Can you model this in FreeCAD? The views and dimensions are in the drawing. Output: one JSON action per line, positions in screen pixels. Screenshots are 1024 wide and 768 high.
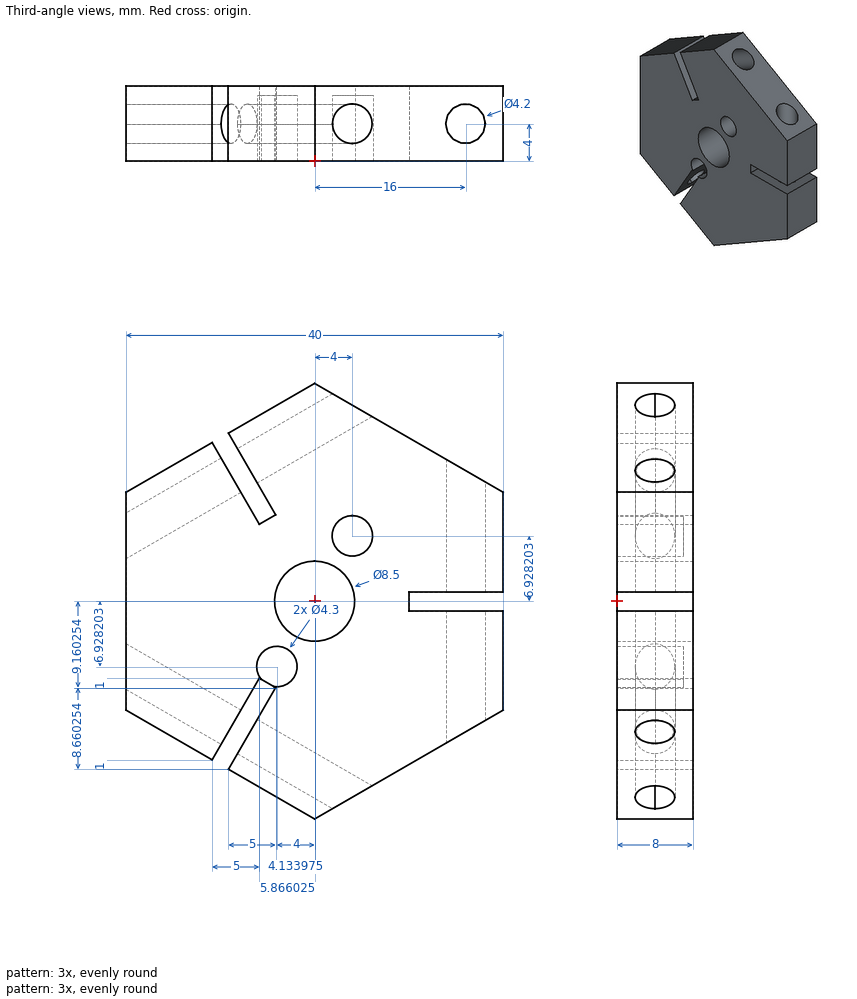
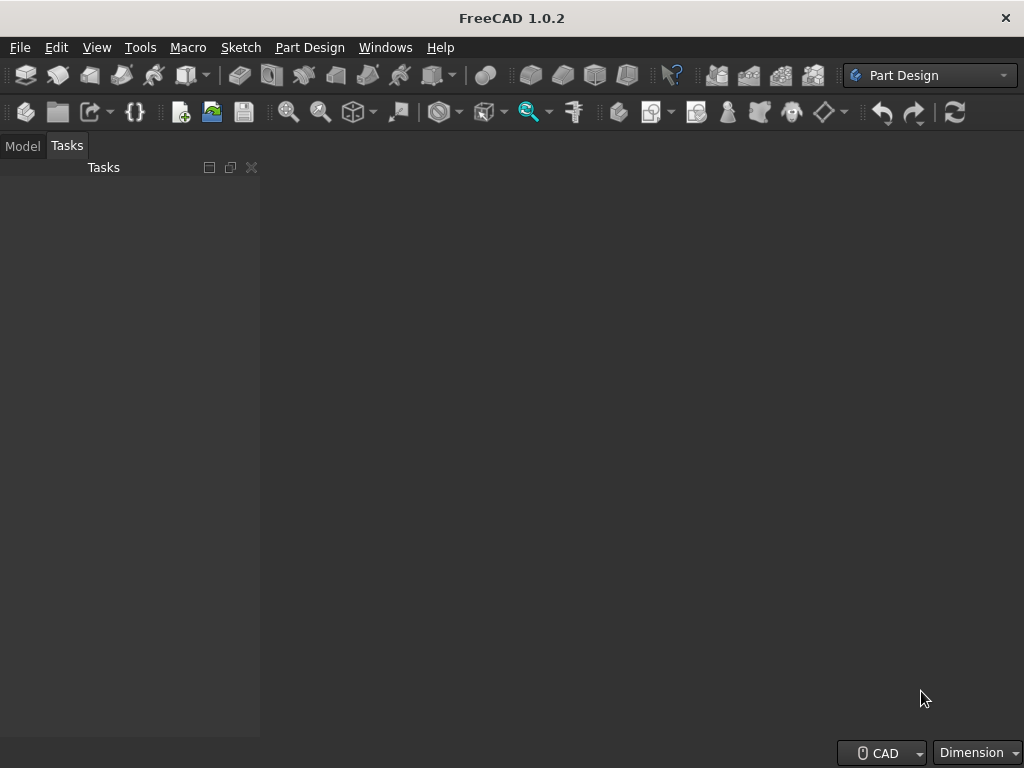
{"action": "left_click", "coordinate": [180, 112]}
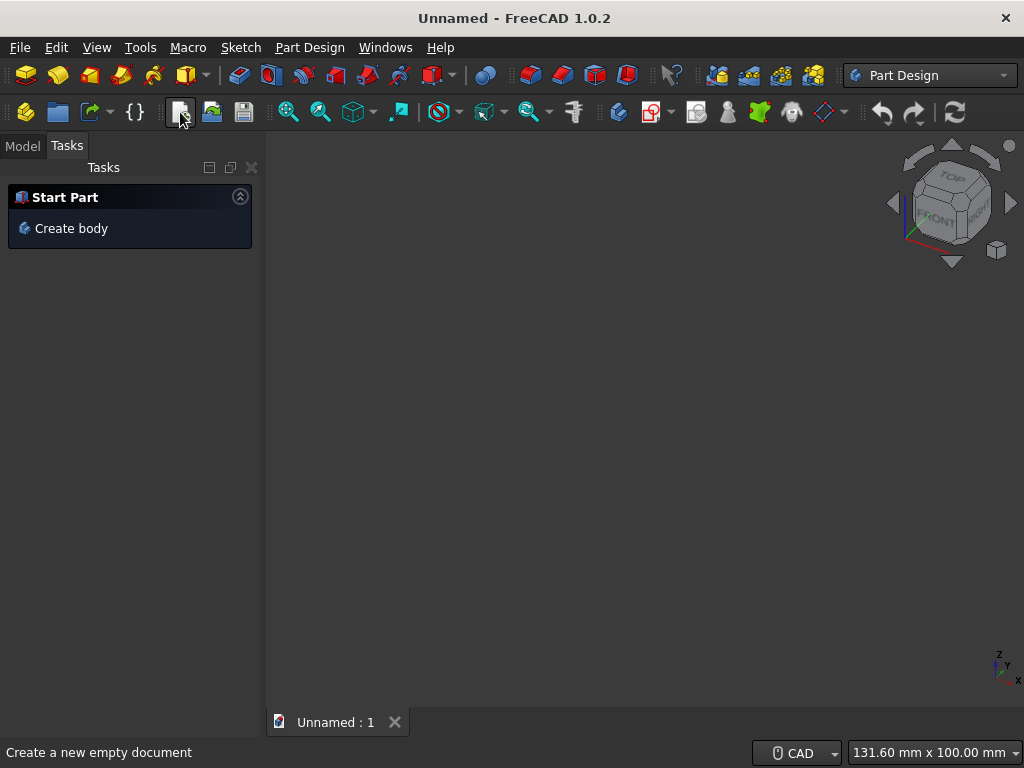
{"action": "left_click", "coordinate": [652, 112]}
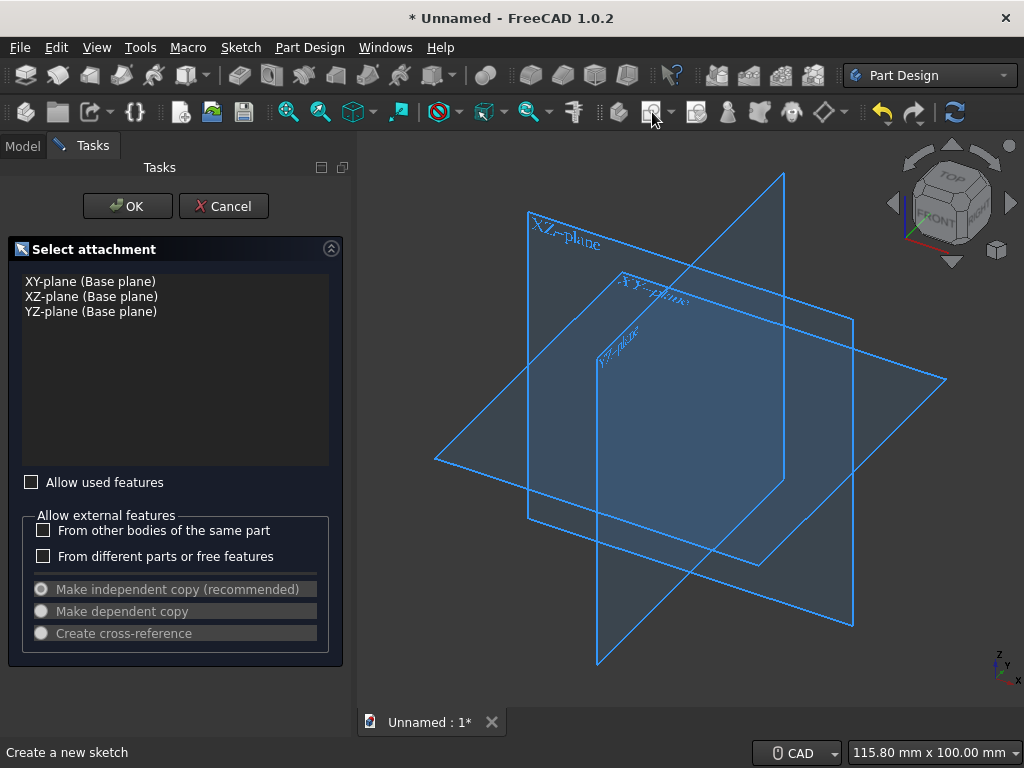
{"action": "left_click", "coordinate": [82, 296]}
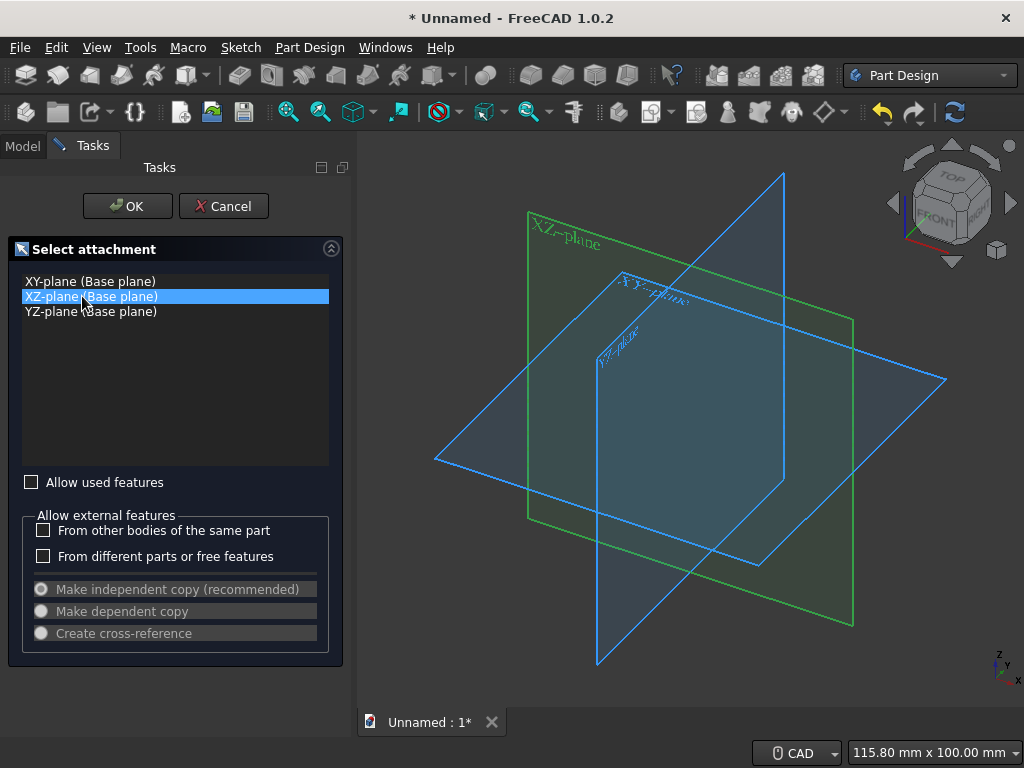
{"action": "left_click", "coordinate": [128, 206]}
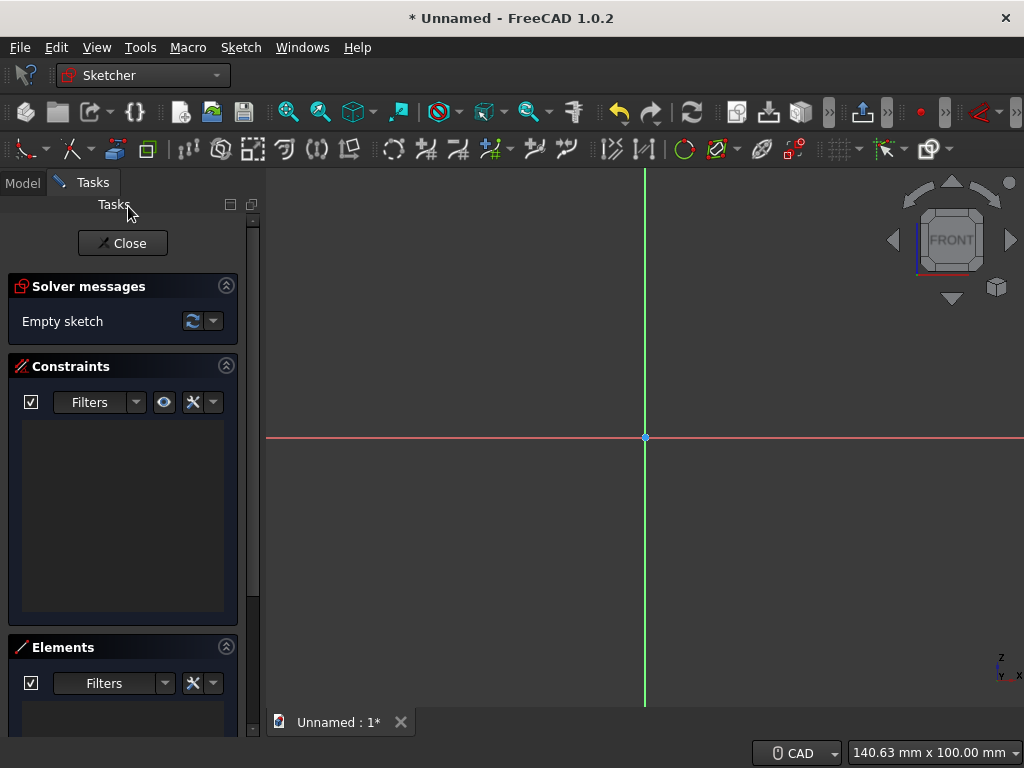
{"action": "scroll", "coordinate": [784, 438], "scroll_direction": "up", "scroll_amount": 2}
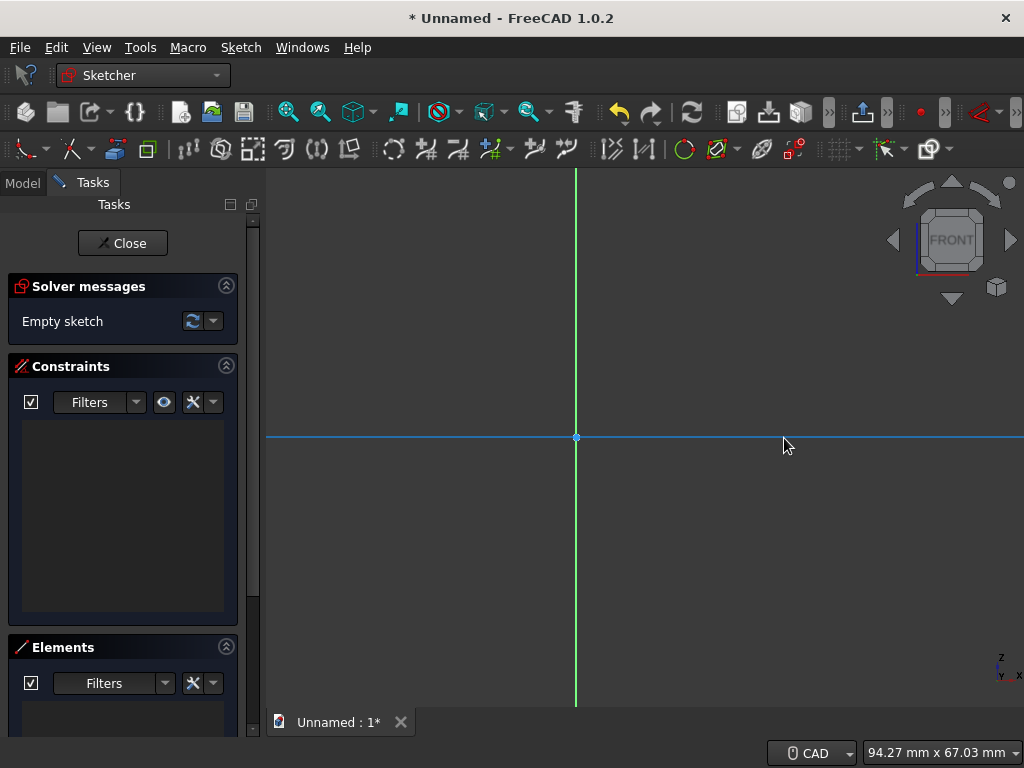
{"action": "key", "text": "g p 6"}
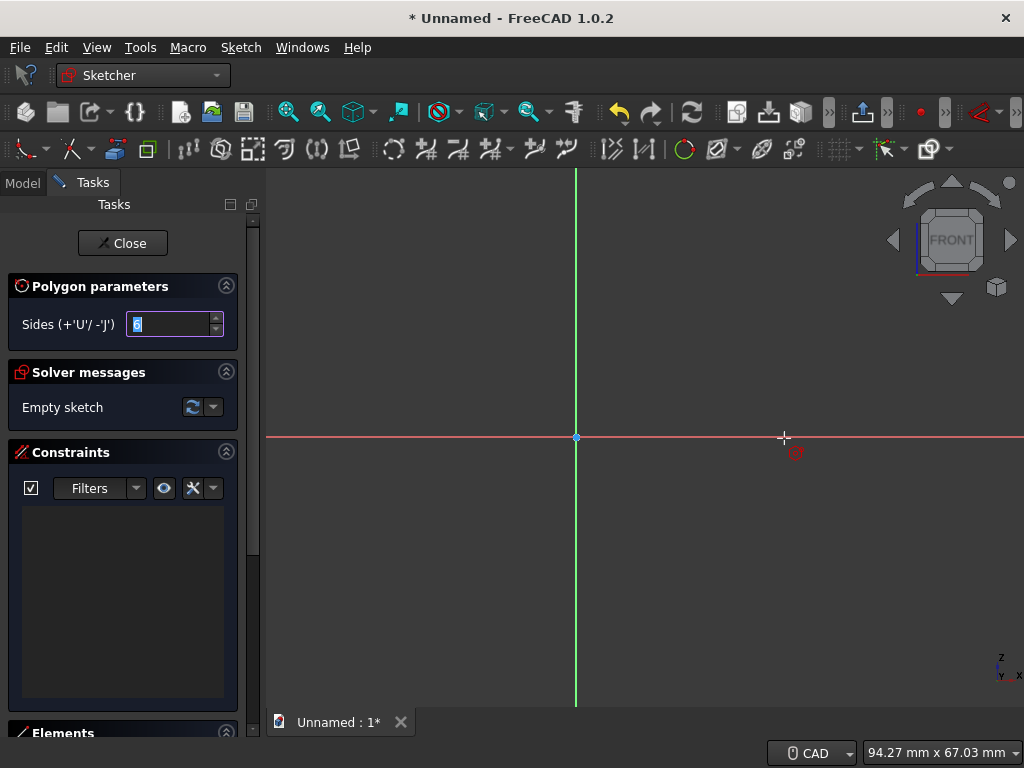
{"action": "left_click", "coordinate": [576, 437]}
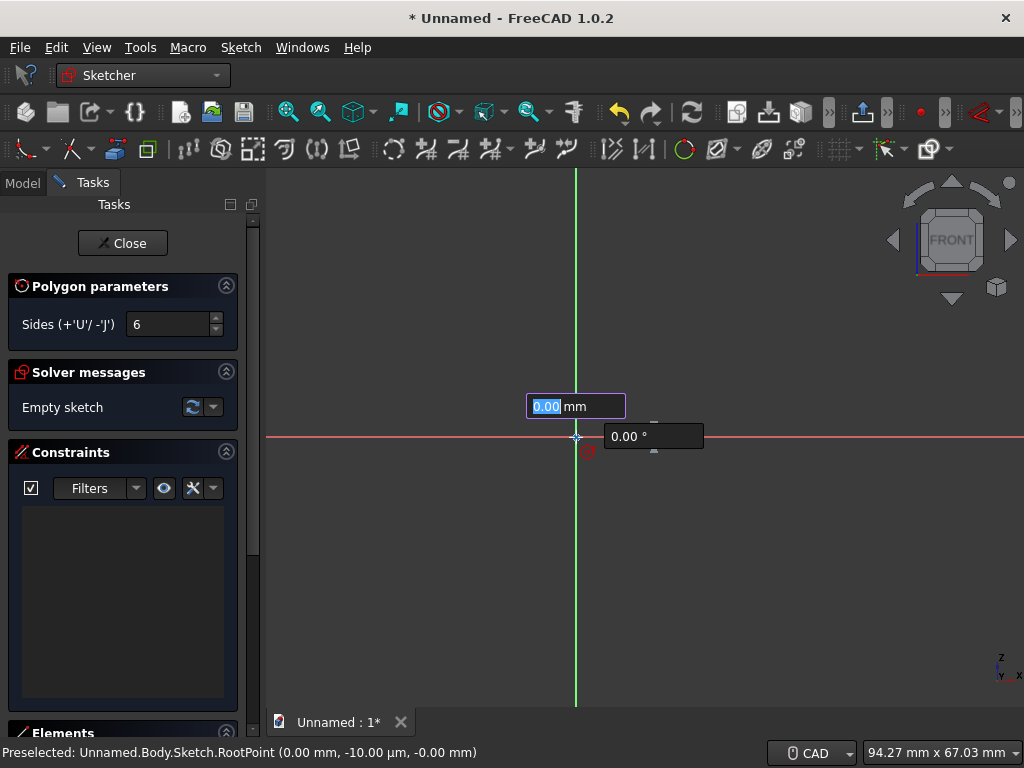
{"action": "left_click", "coordinate": [576, 623]}
{"action": "right_click", "coordinate": [576, 623]}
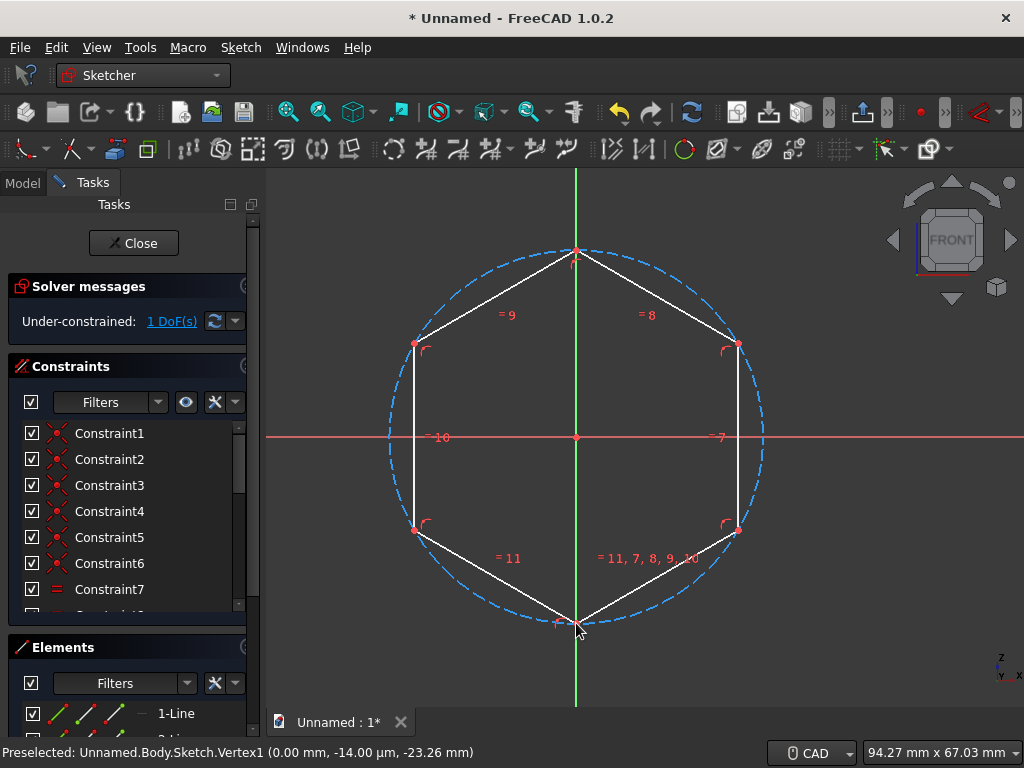
{"action": "left_click", "coordinate": [980, 112]}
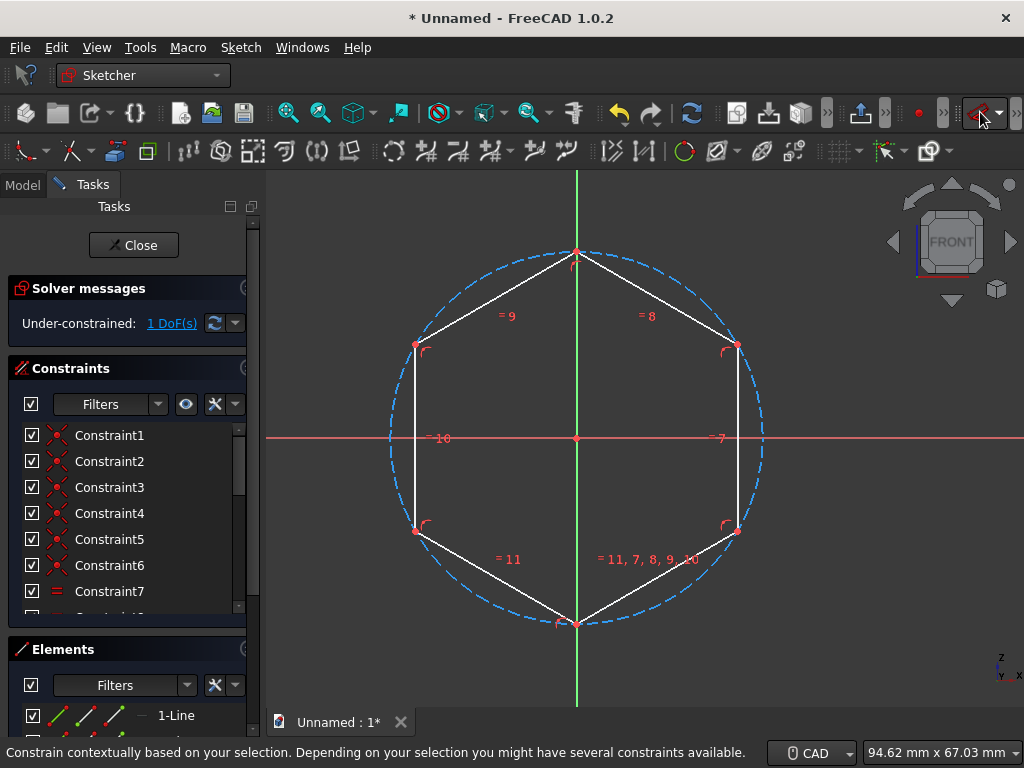
{"action": "left_click", "coordinate": [415, 345]}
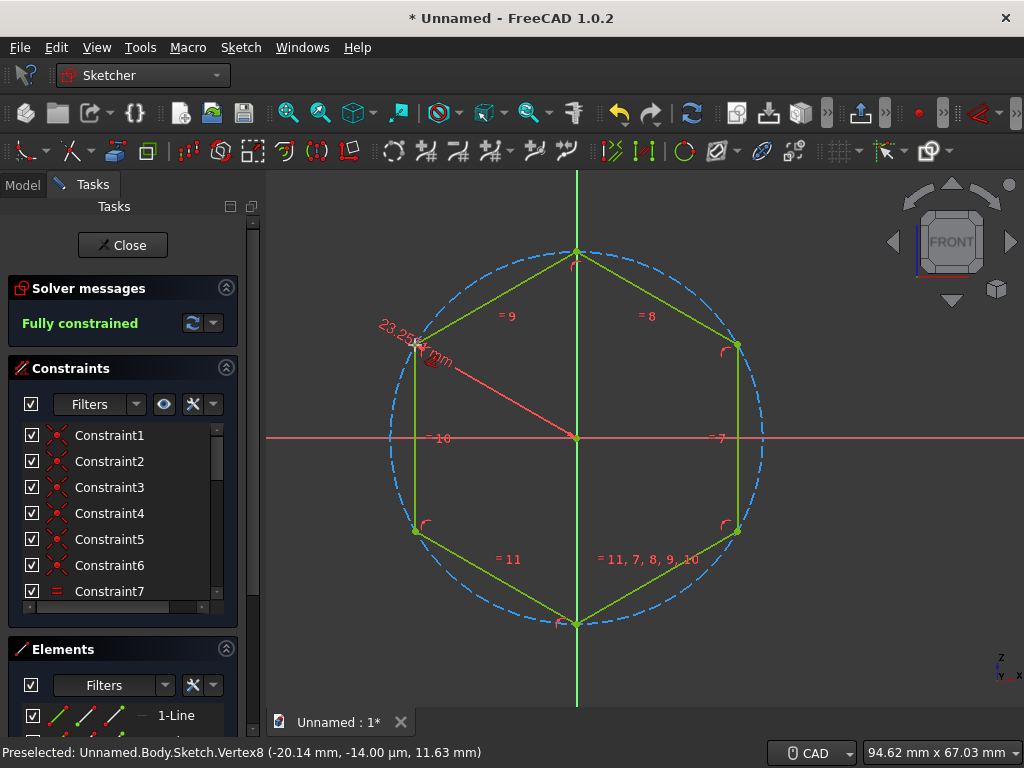
{"action": "left_click", "coordinate": [738, 531]}
{"action": "left_click", "coordinate": [502, 565]}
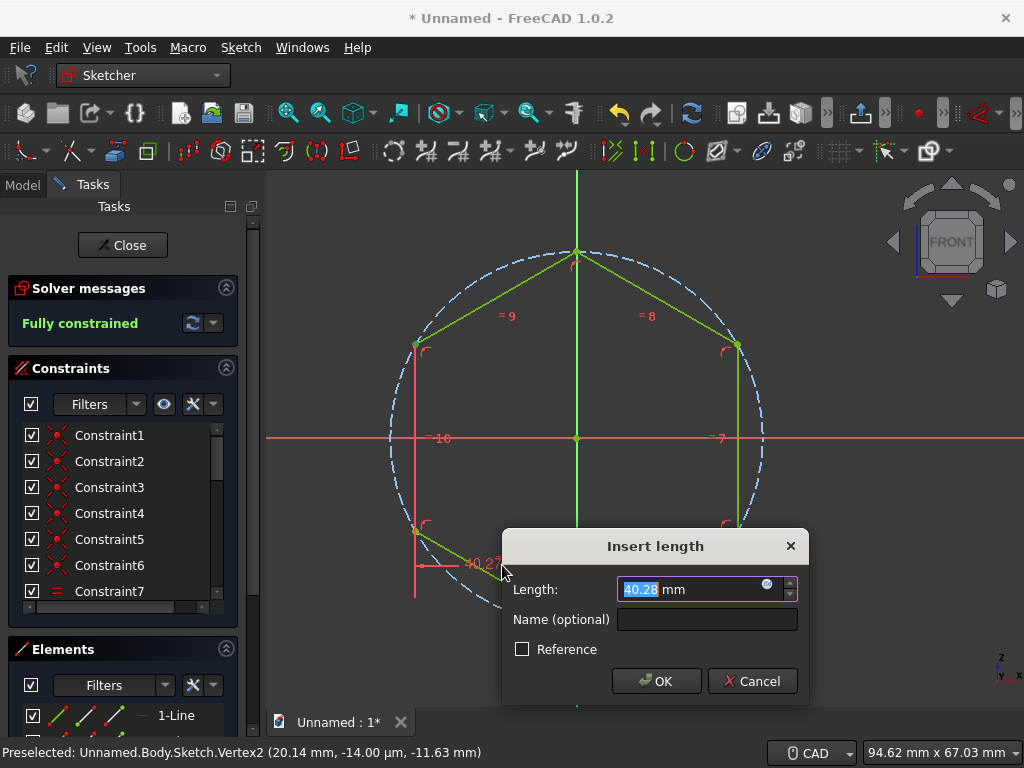
{"action": "type", "text": "40"}
{"action": "key", "text": "Return"}
{"action": "key", "text": "Escape"}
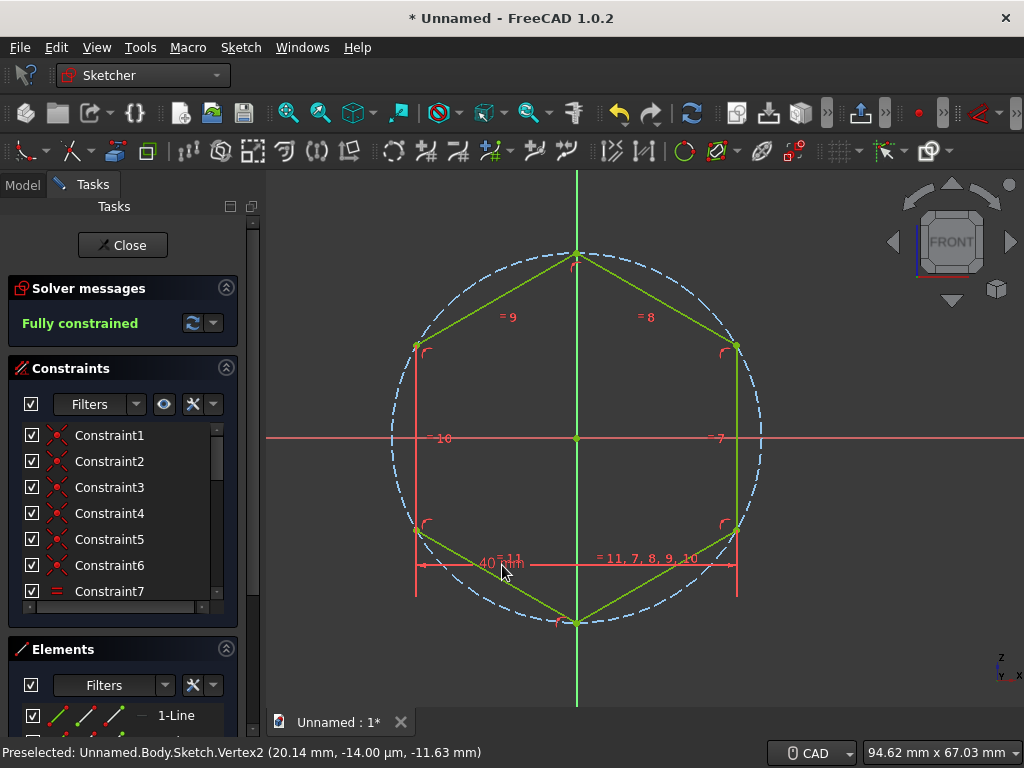
{"action": "left_click", "coordinate": [123, 245]}